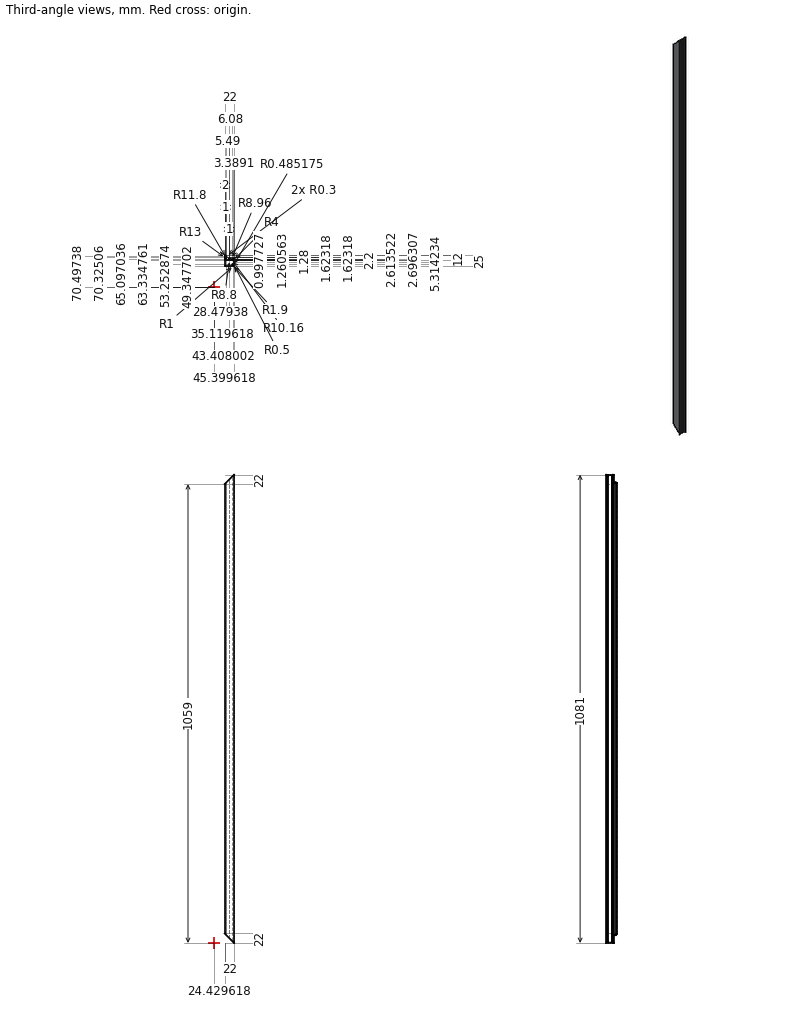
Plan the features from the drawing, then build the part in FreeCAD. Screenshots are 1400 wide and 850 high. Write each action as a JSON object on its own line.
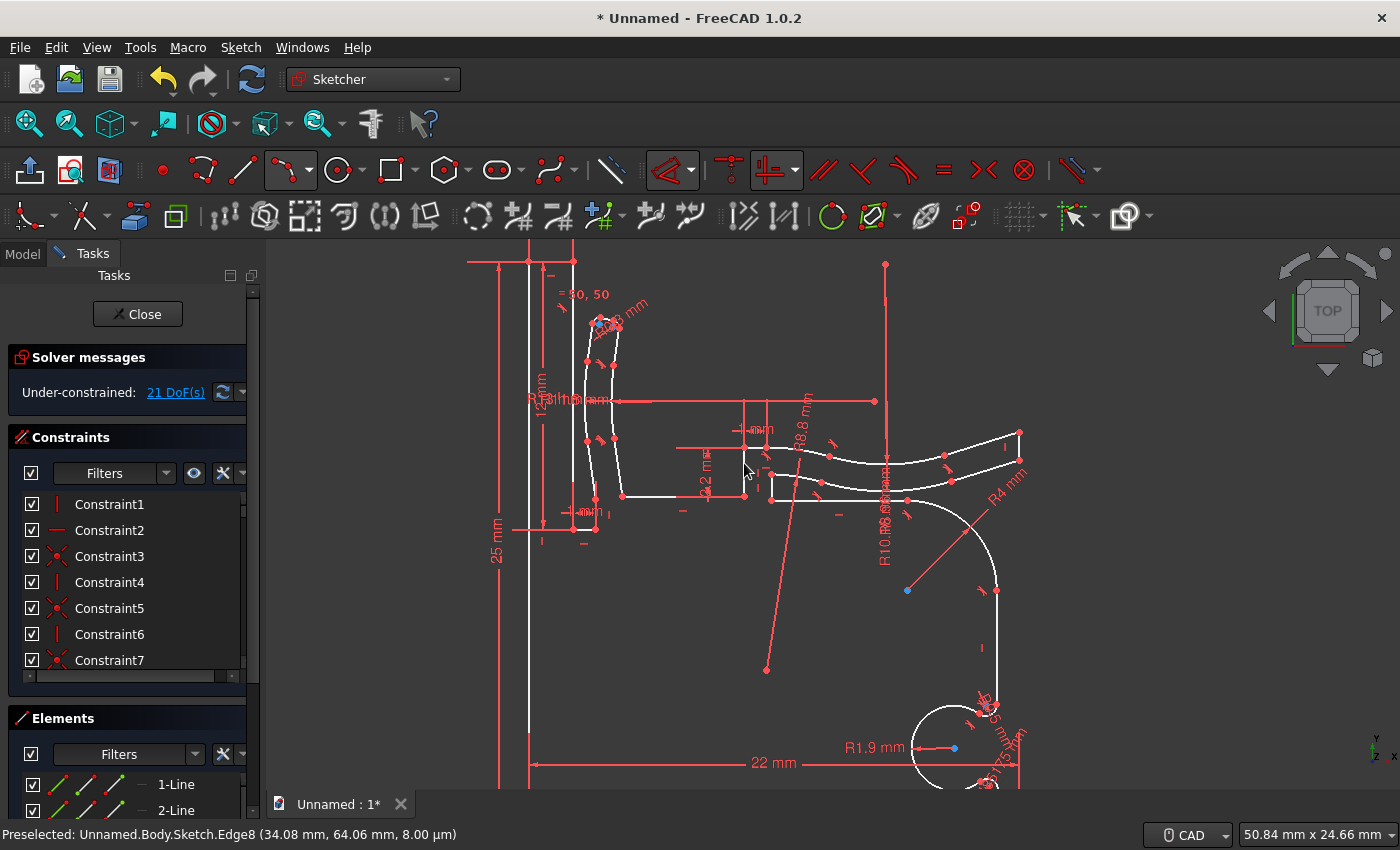
{"action": "scroll", "coordinate": [867, 501], "scroll_direction": "up", "scroll_amount": 2}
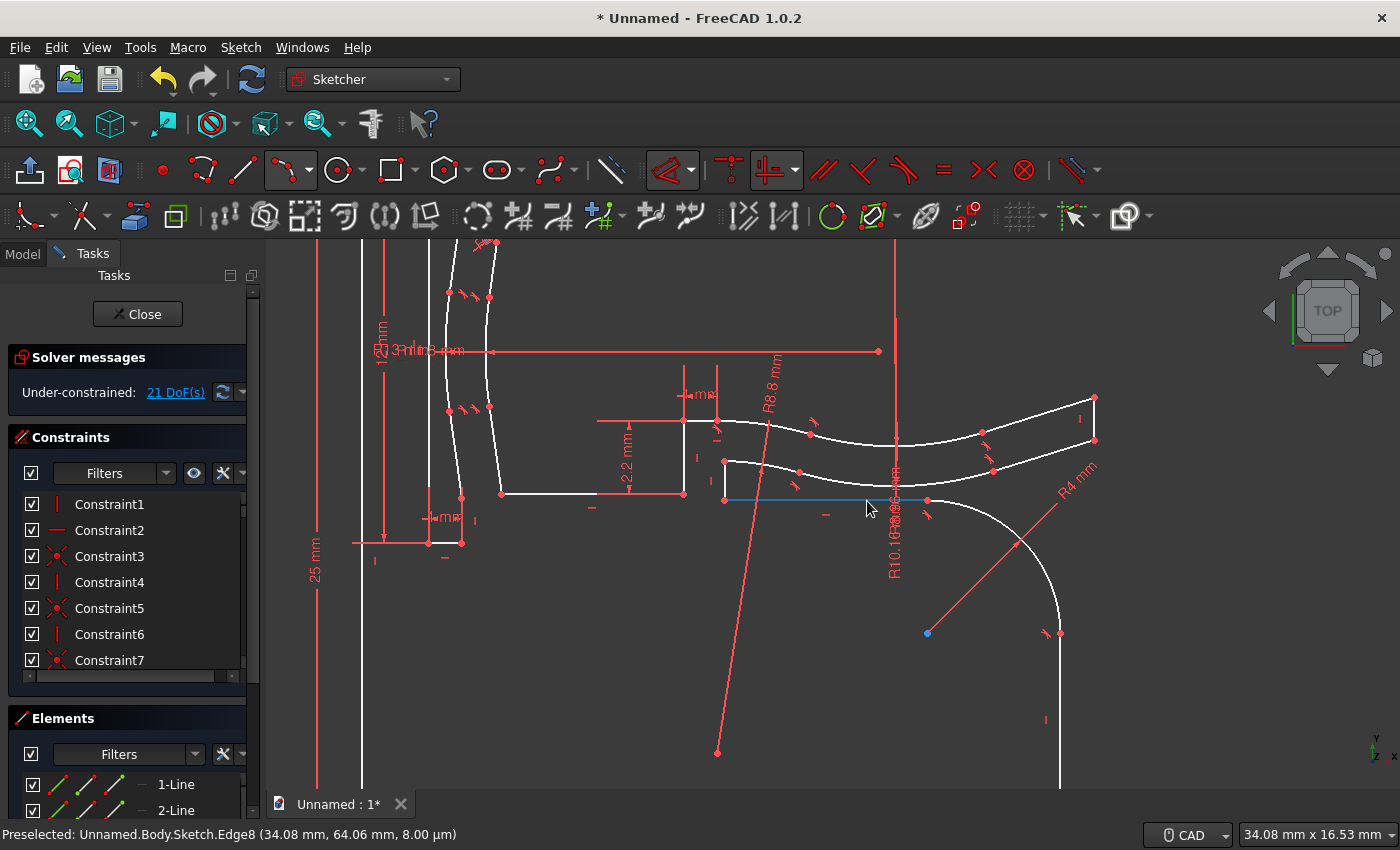
{"action": "left_click", "coordinate": [867, 500]}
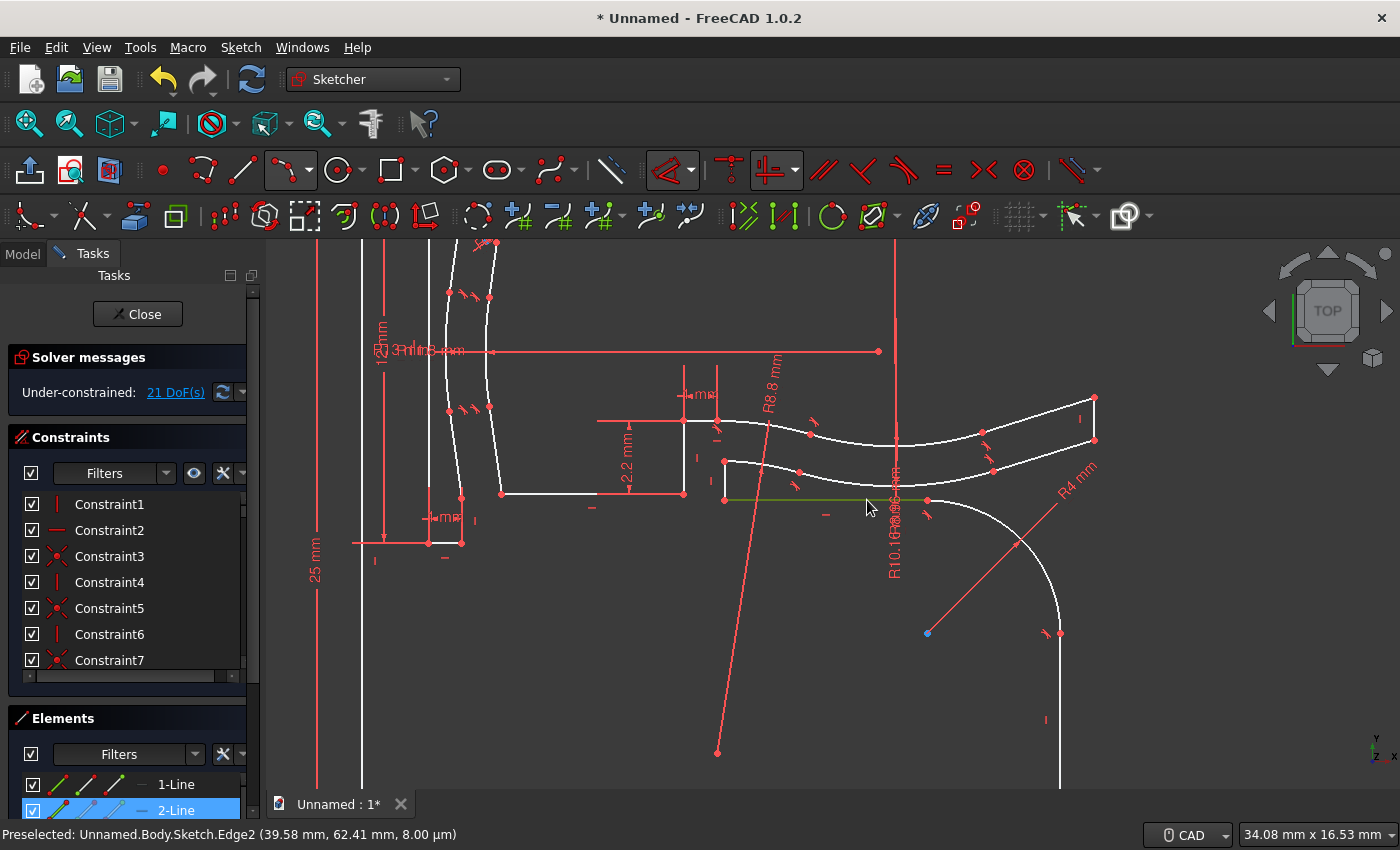
{"action": "left_click", "coordinate": [694, 170]}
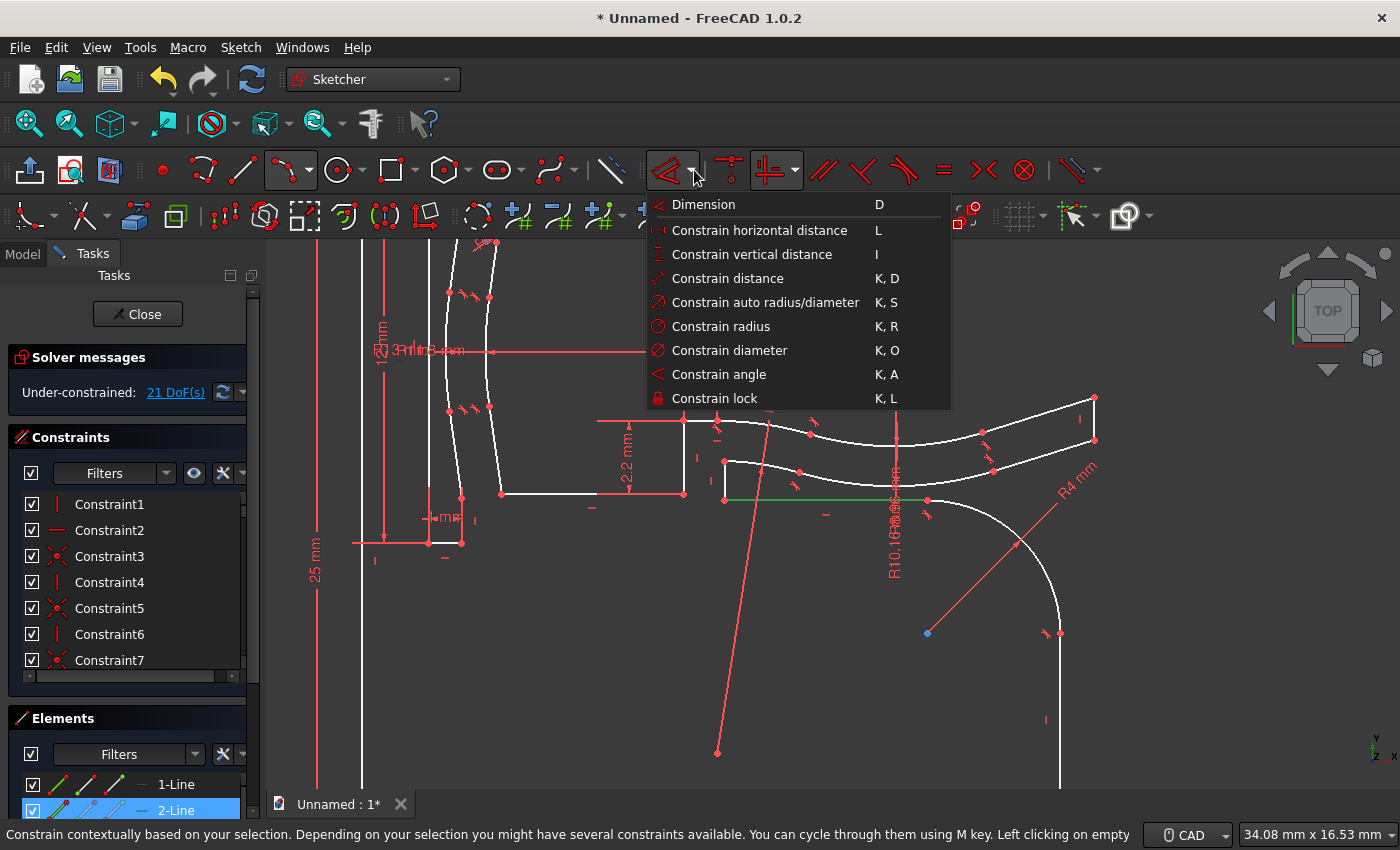
{"action": "left_click", "coordinate": [799, 230]}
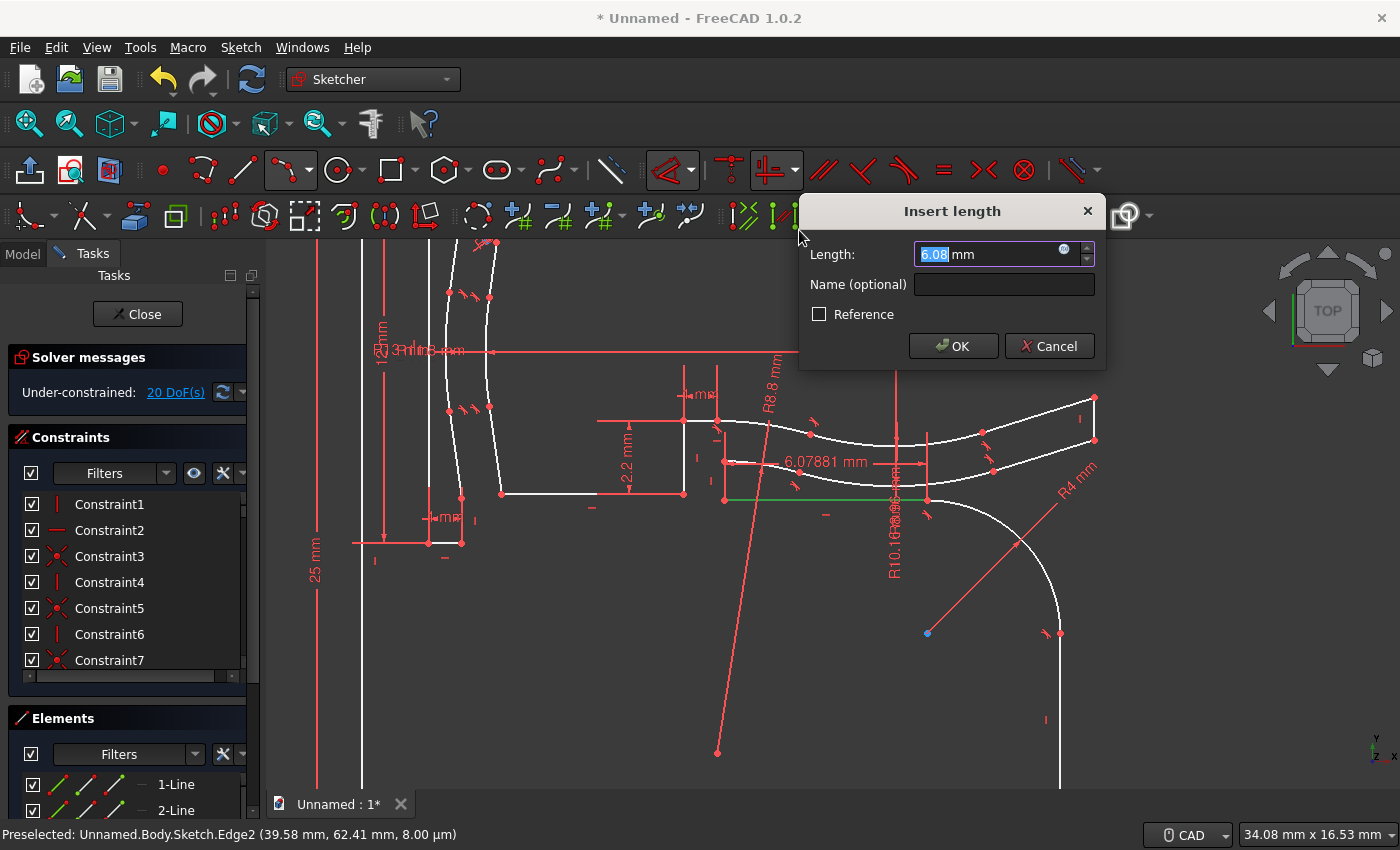
{"action": "type", "text": "6.08"}
{"action": "key", "text": "Return"}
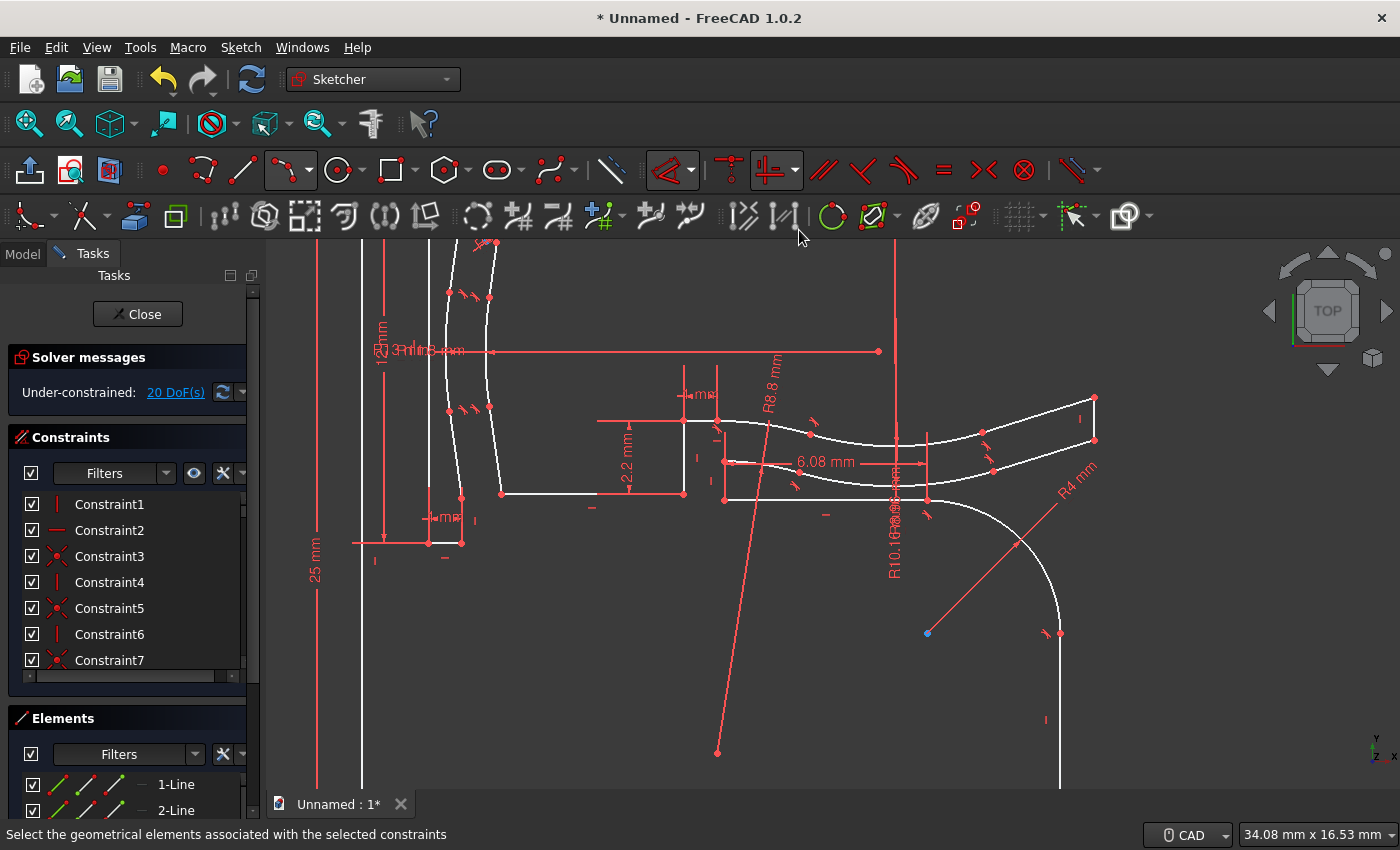
{"action": "left_click", "coordinate": [629, 494]}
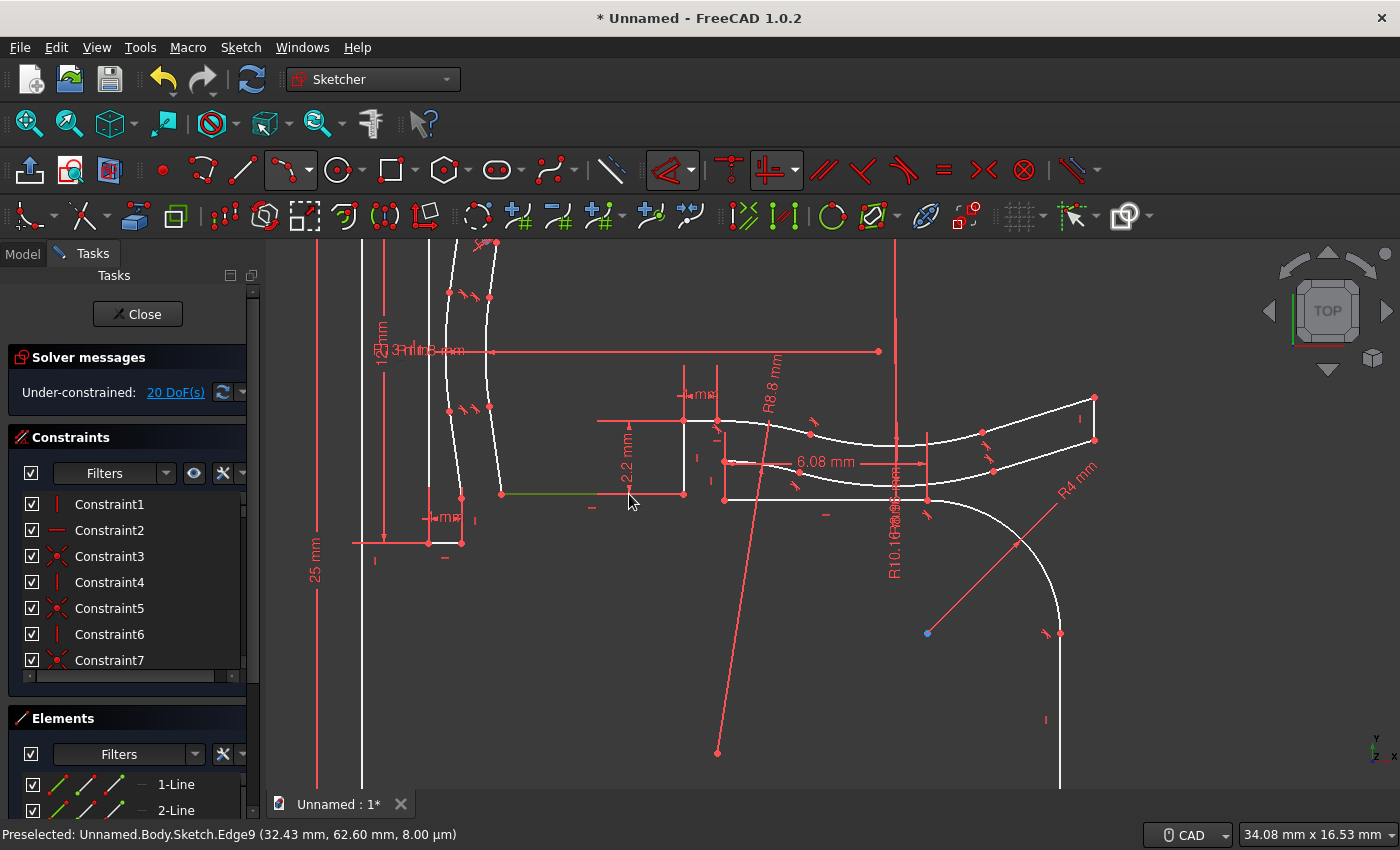
{"action": "key", "text": "l"}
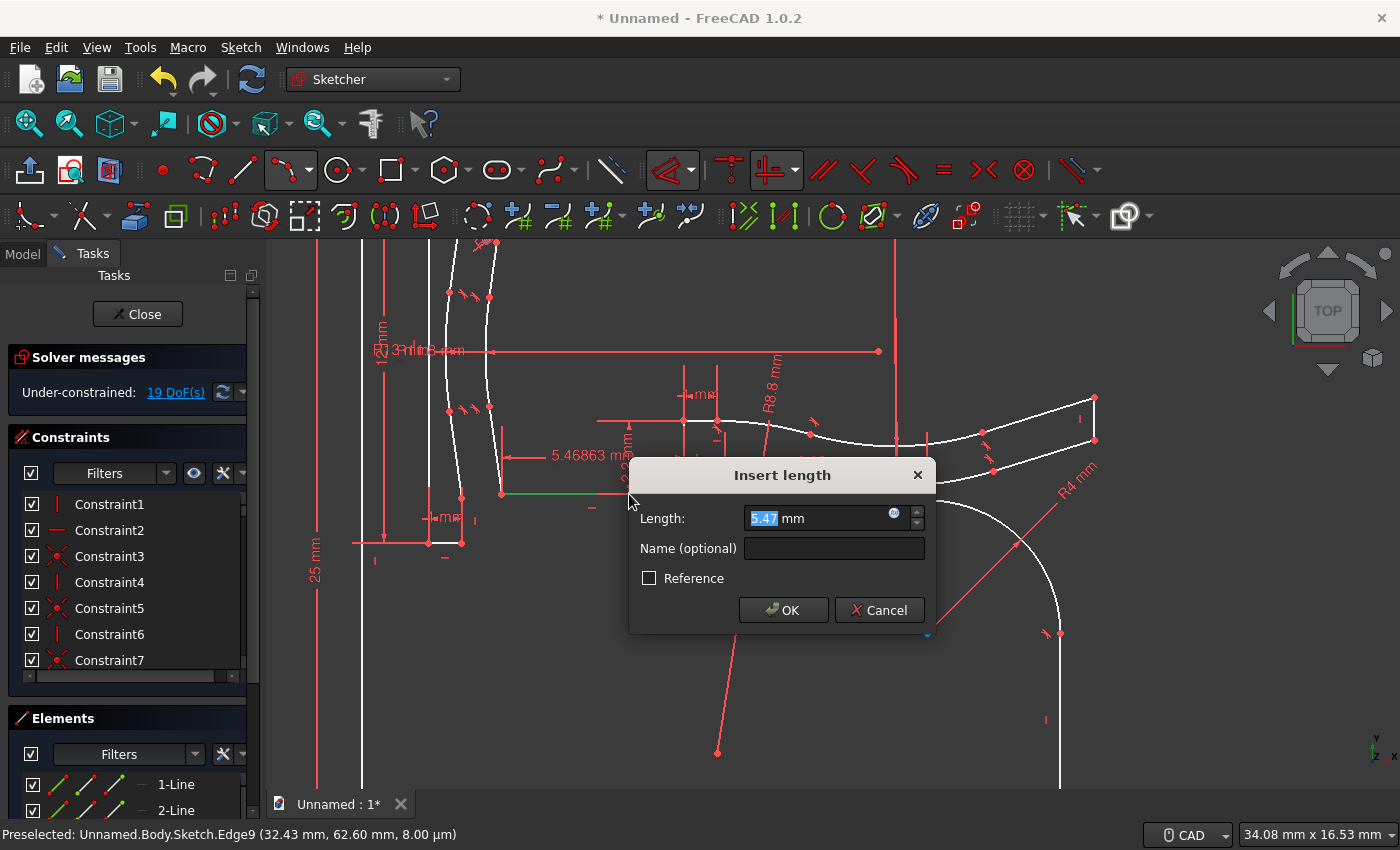
{"action": "type", "text": "5.49"}
{"action": "key", "text": "Return"}